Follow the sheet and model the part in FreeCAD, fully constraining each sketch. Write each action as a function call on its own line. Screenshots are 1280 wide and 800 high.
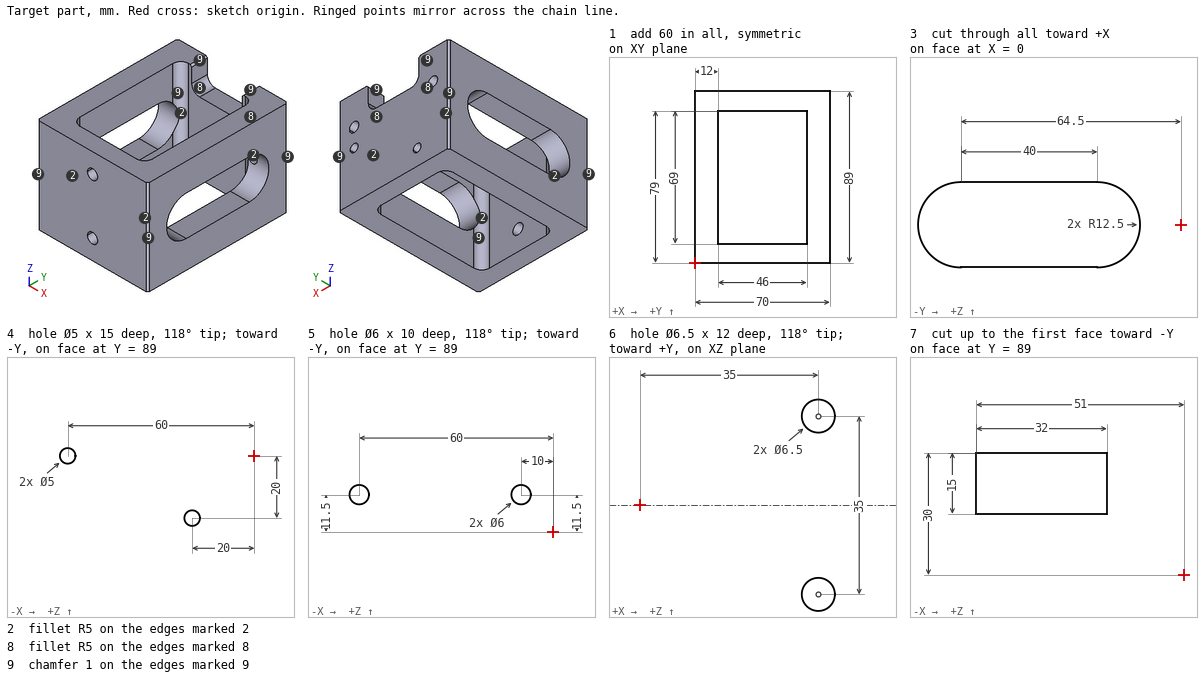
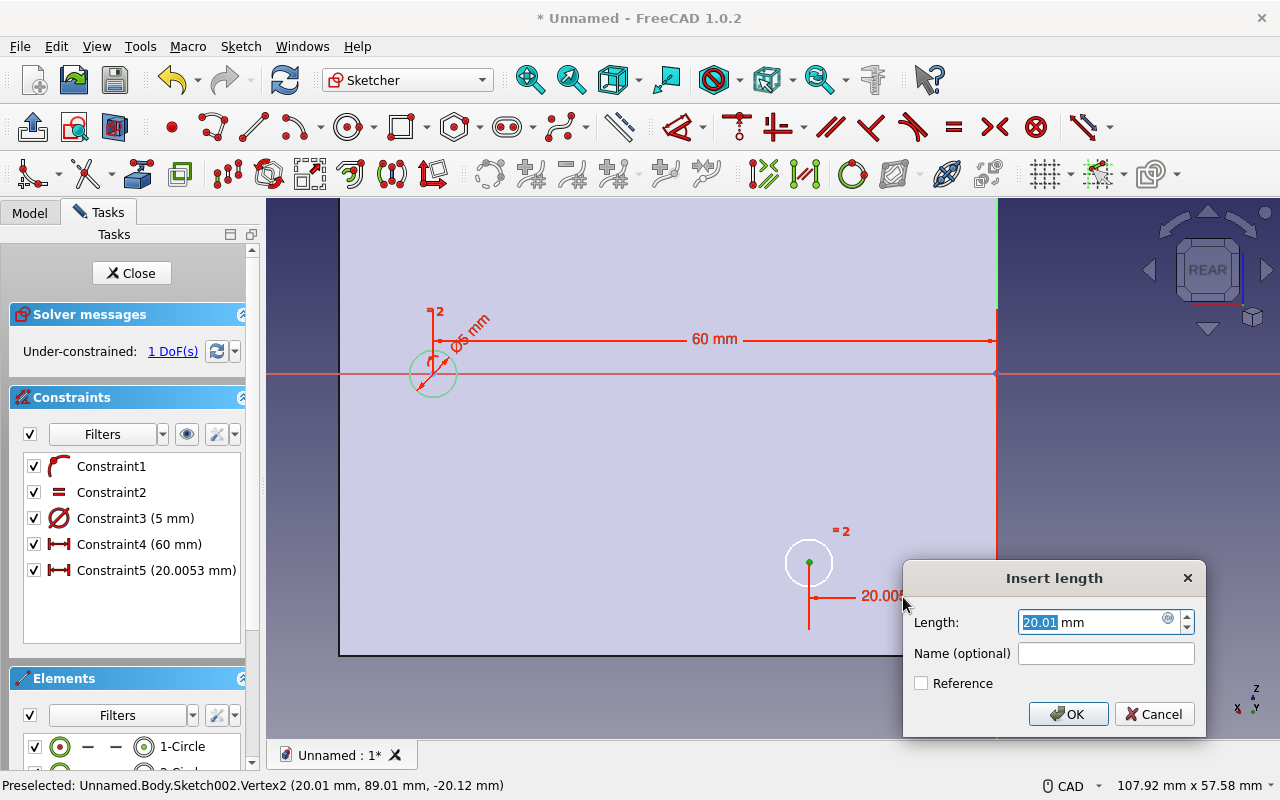
text(20)
key(Return)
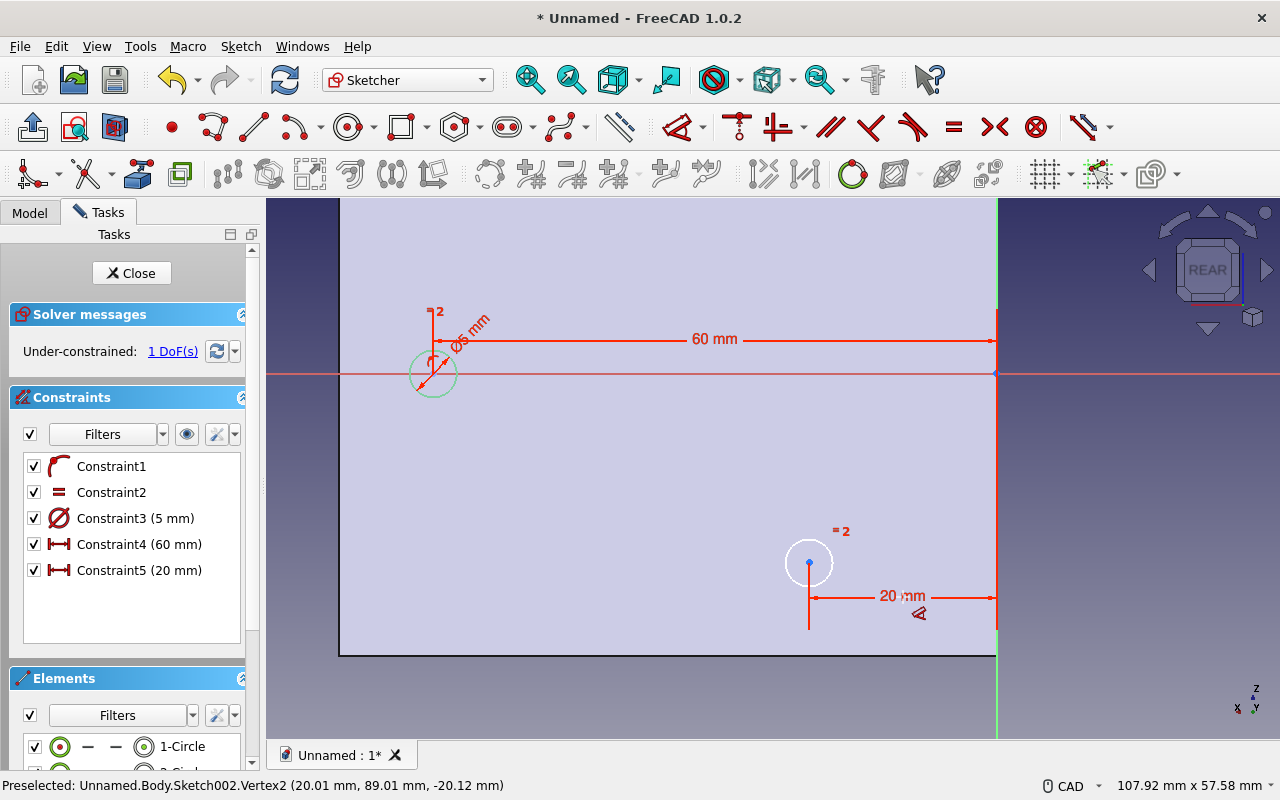
click(809, 563)
click(1031, 468)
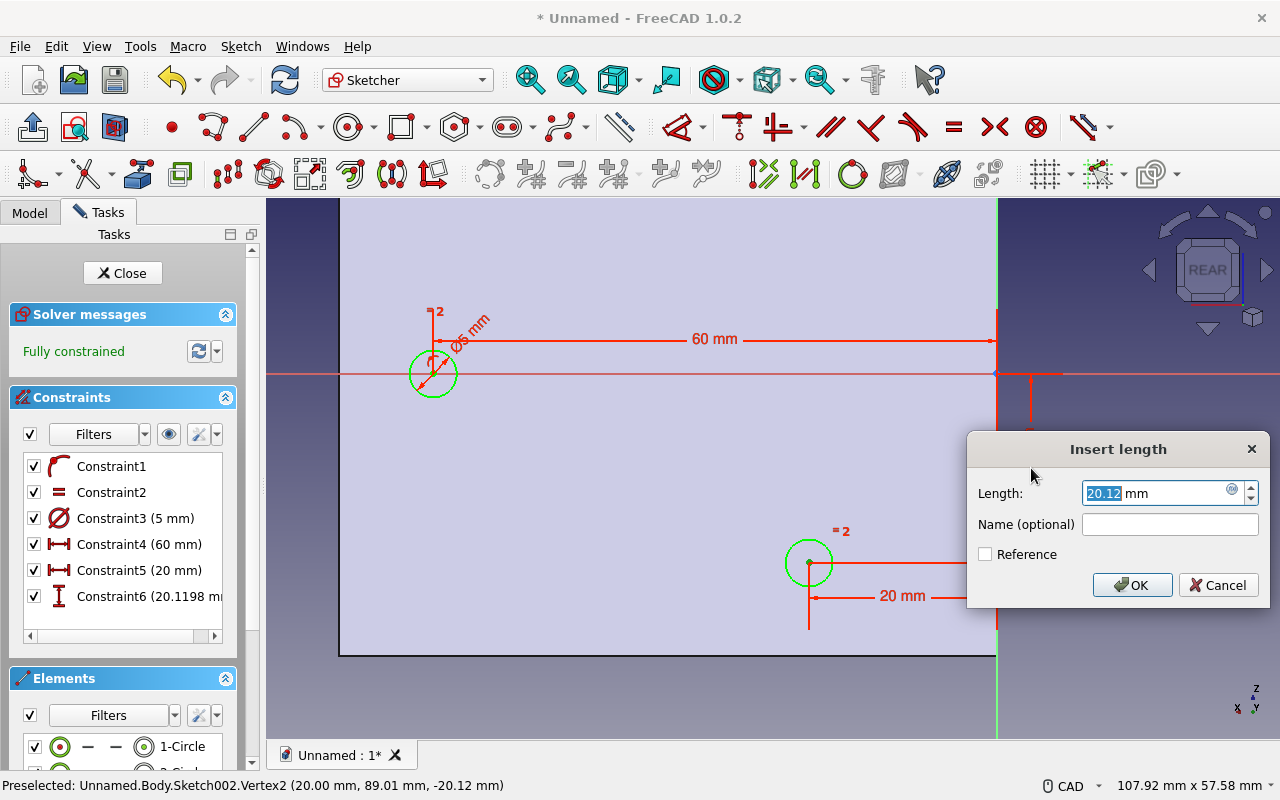
text(20)
key(Return)
key(Escape)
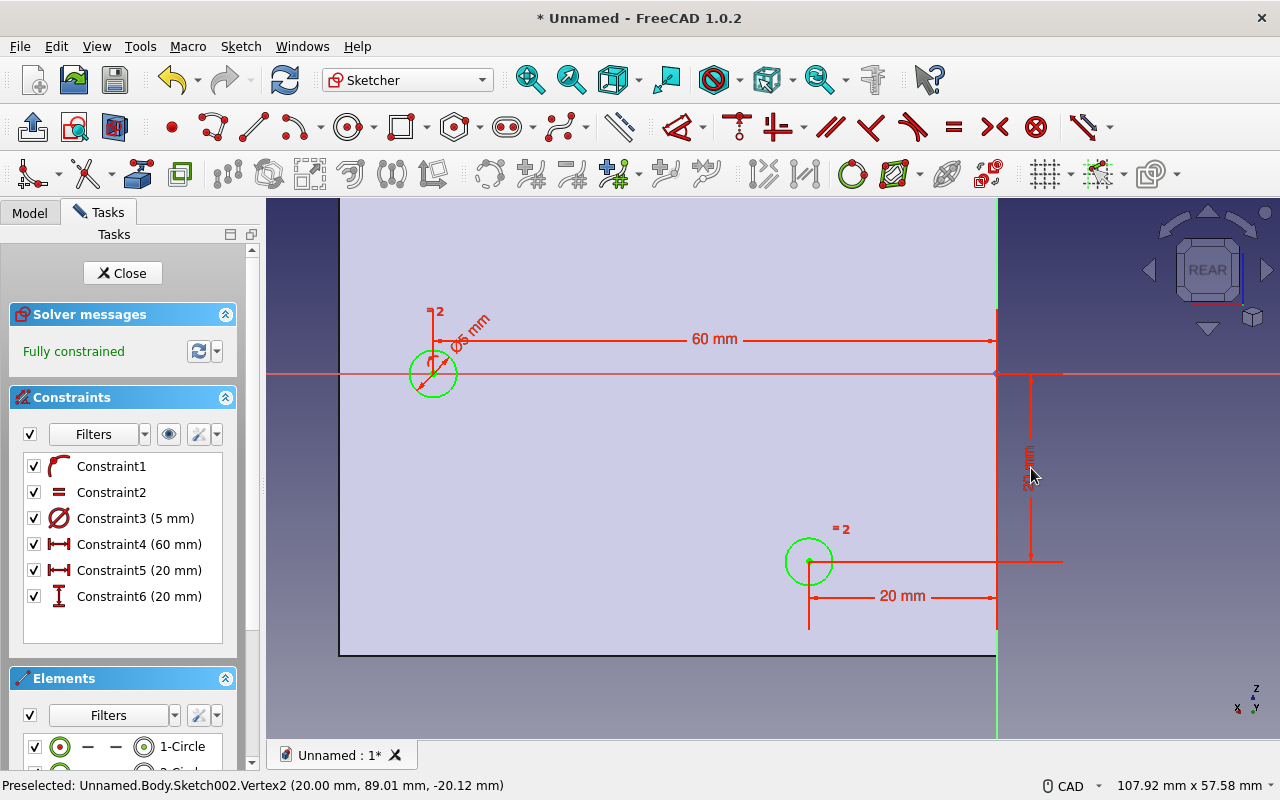
click(123, 273)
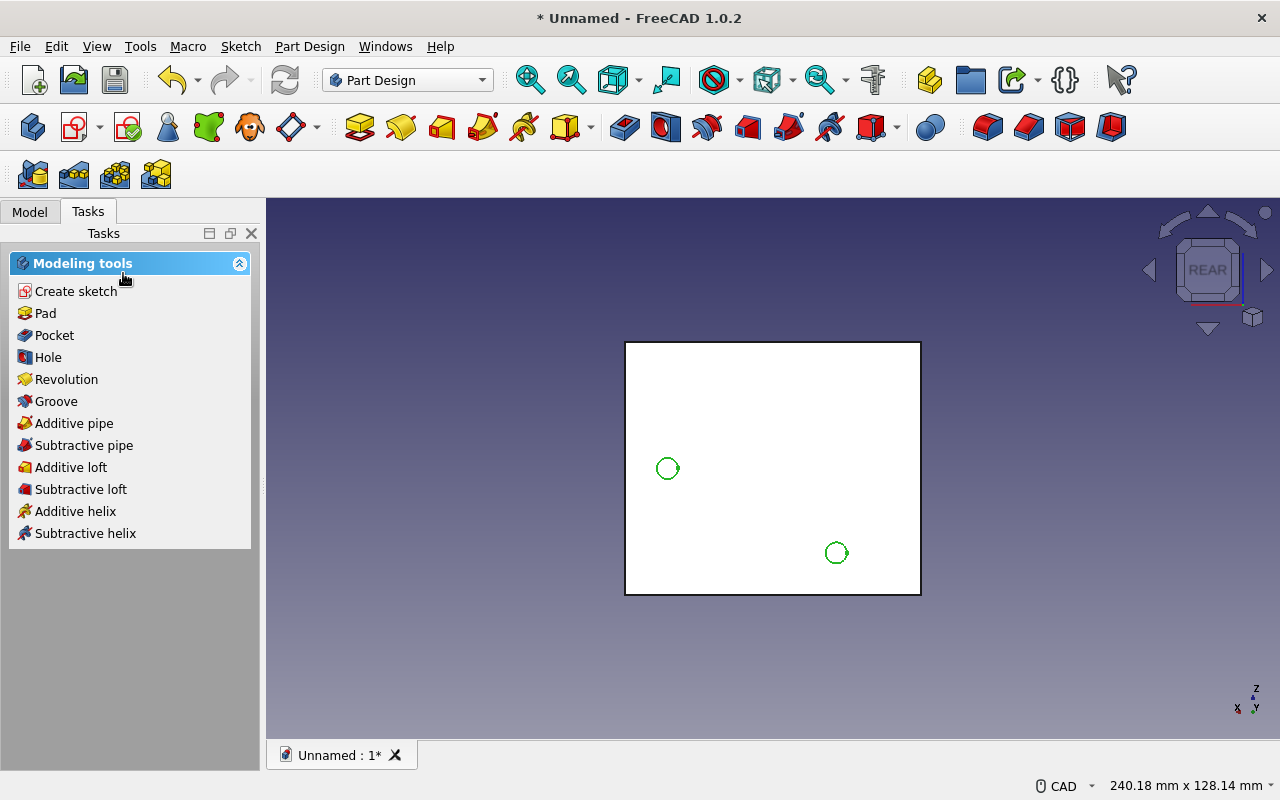
click(666, 128)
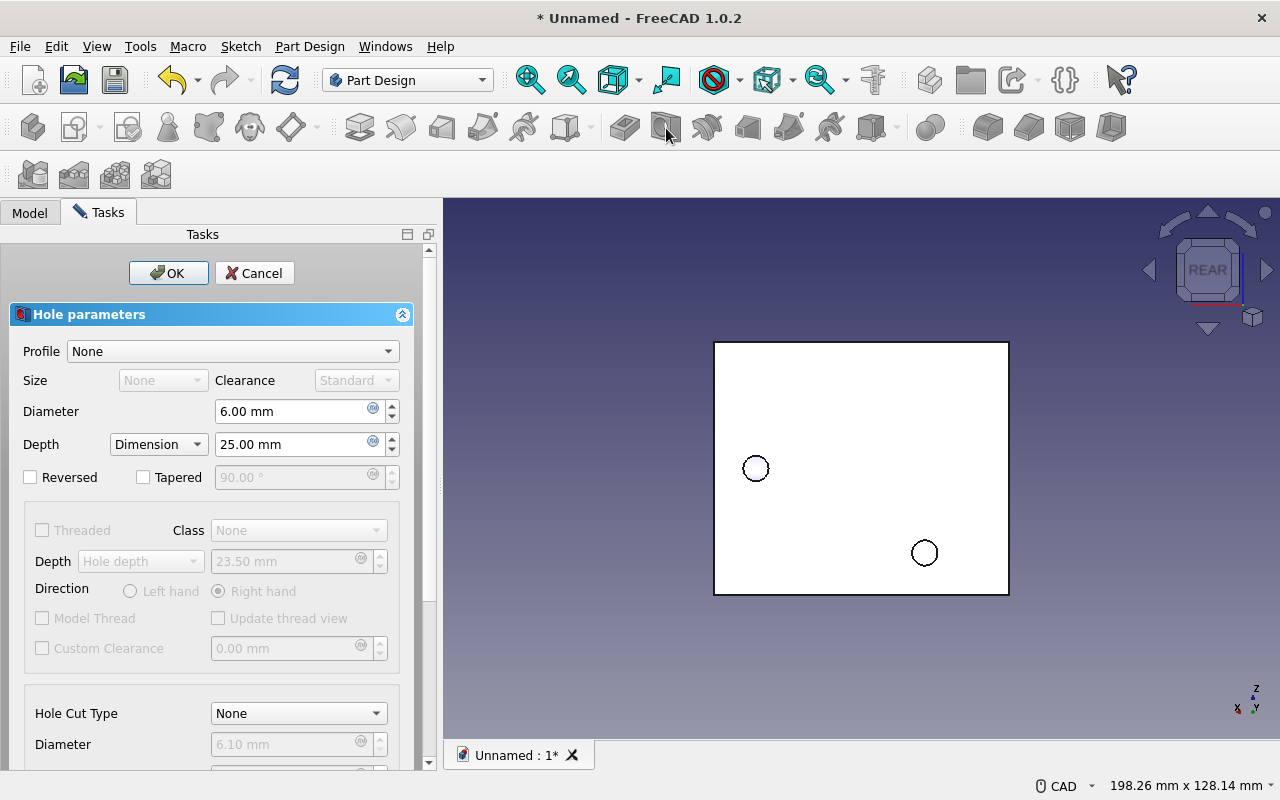
triple_click(300, 412)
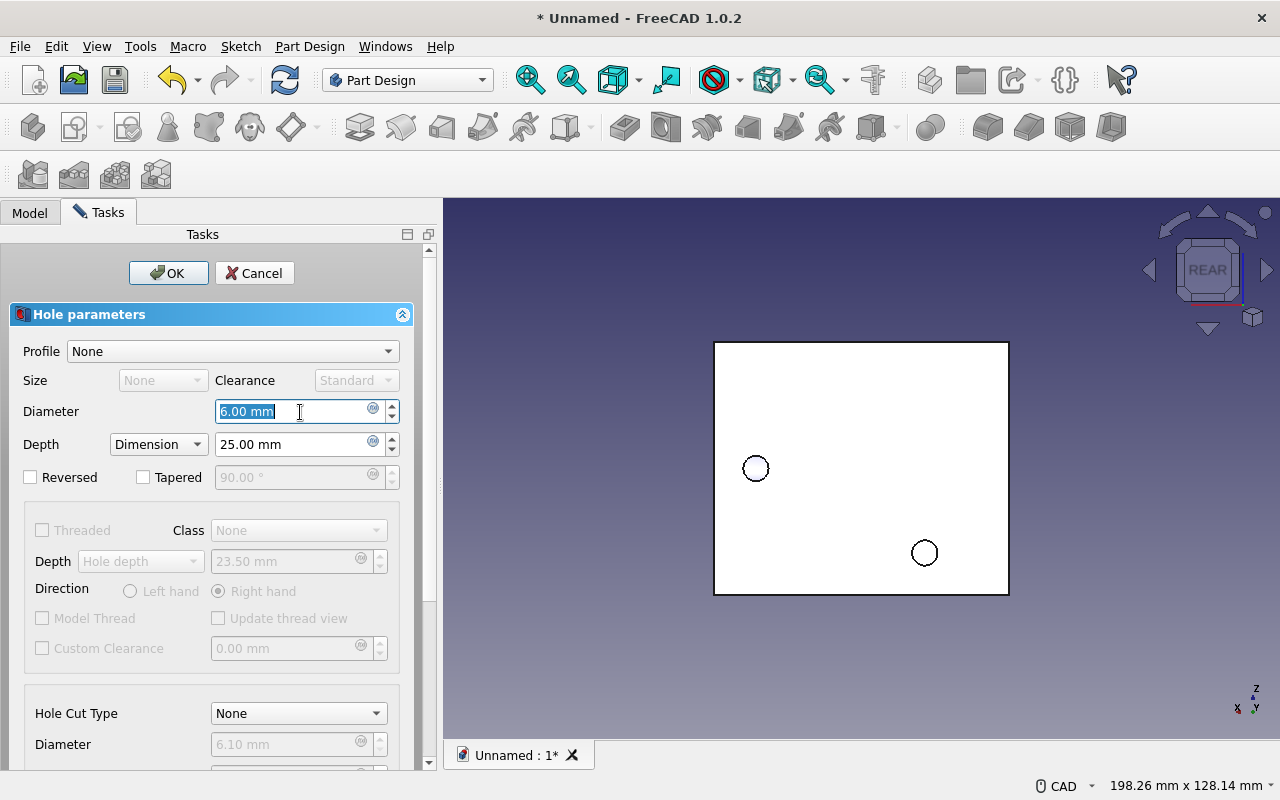
text(5)
key(Tab)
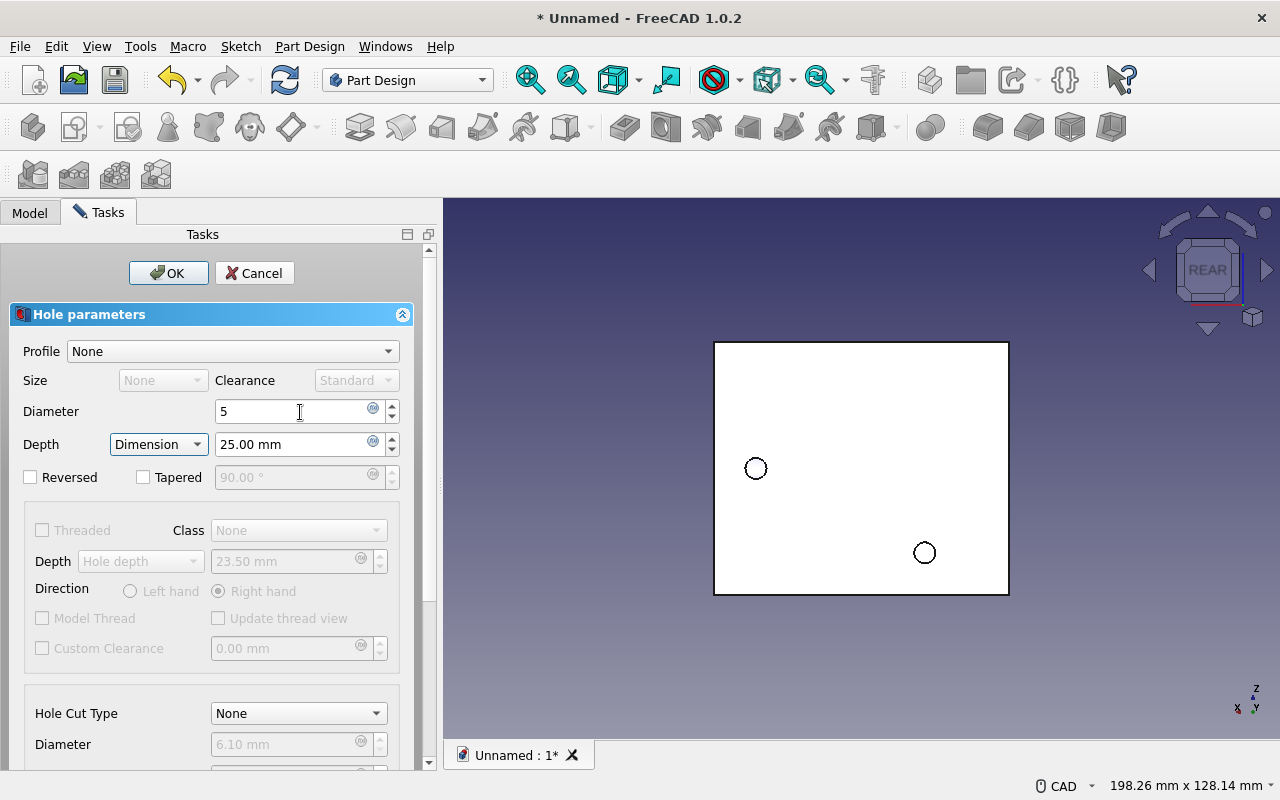
triple_click(300, 444)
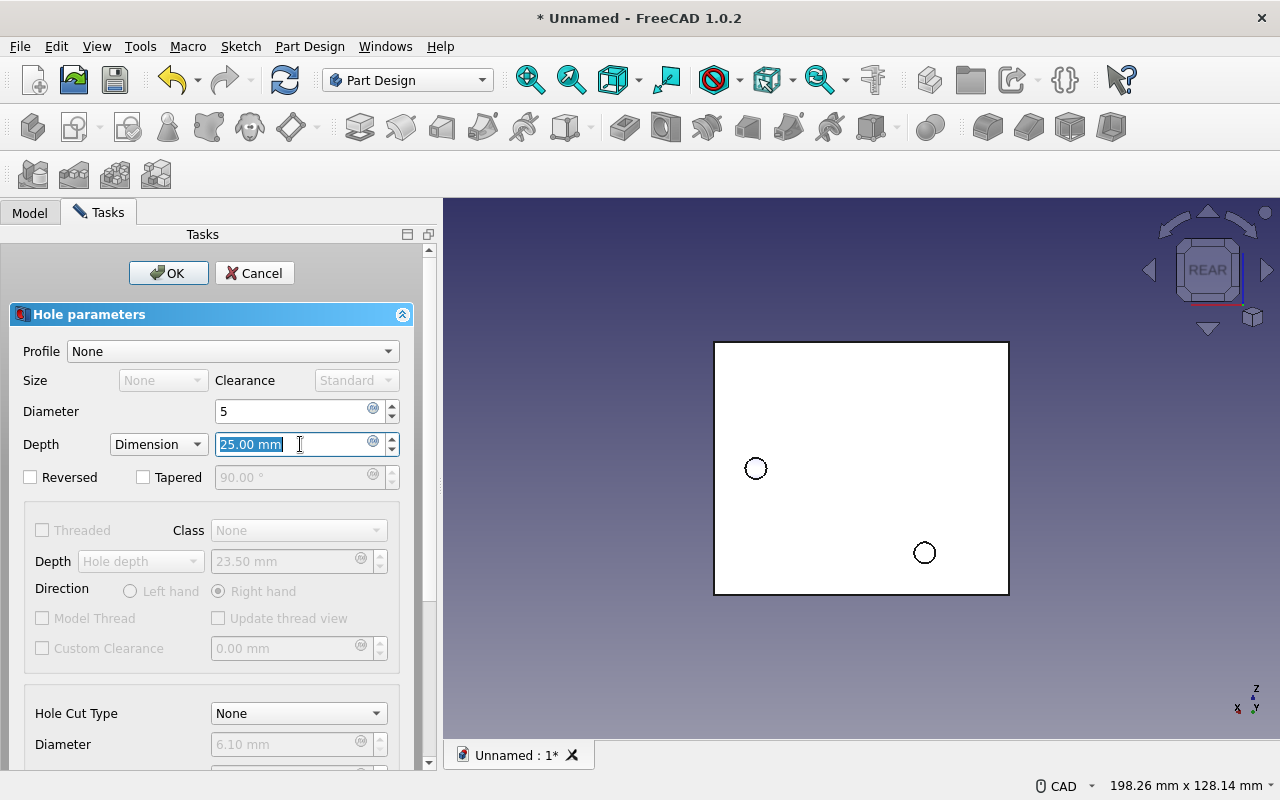
text(15)
key(Tab)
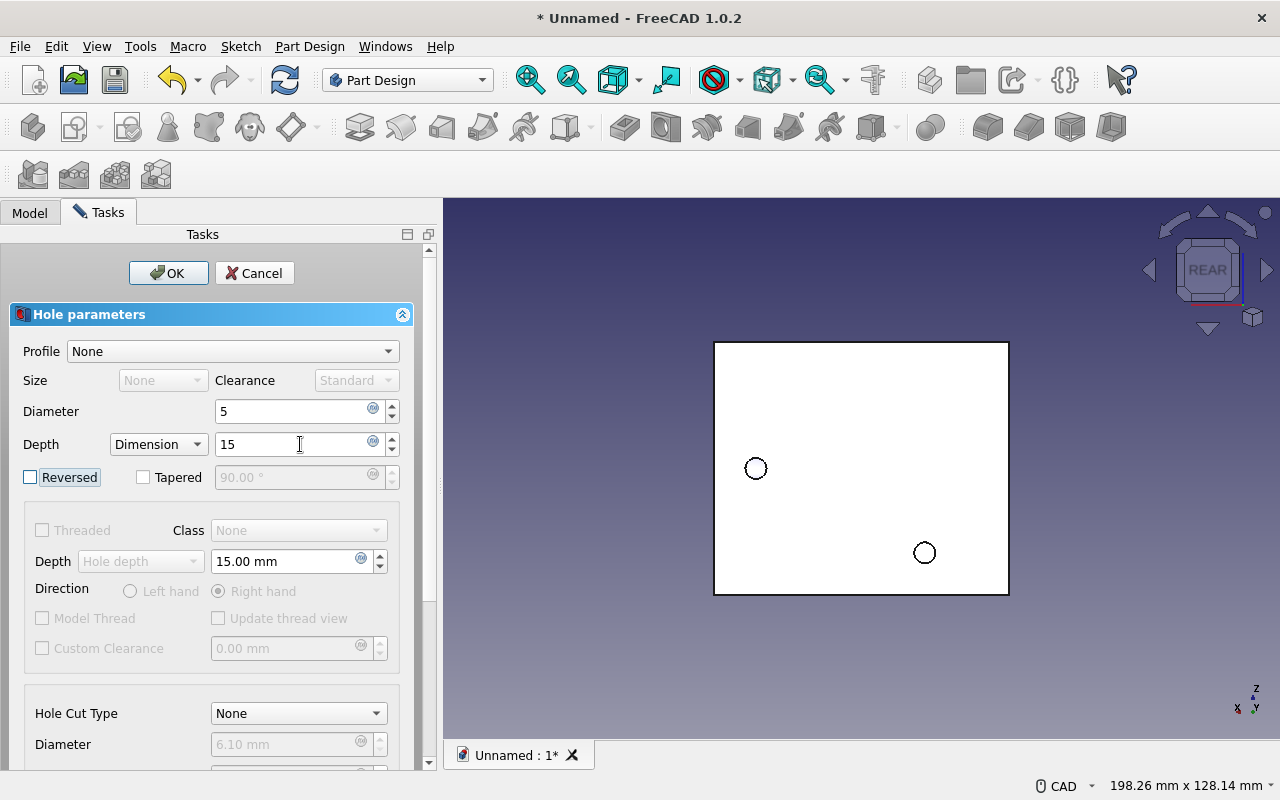
click(169, 273)